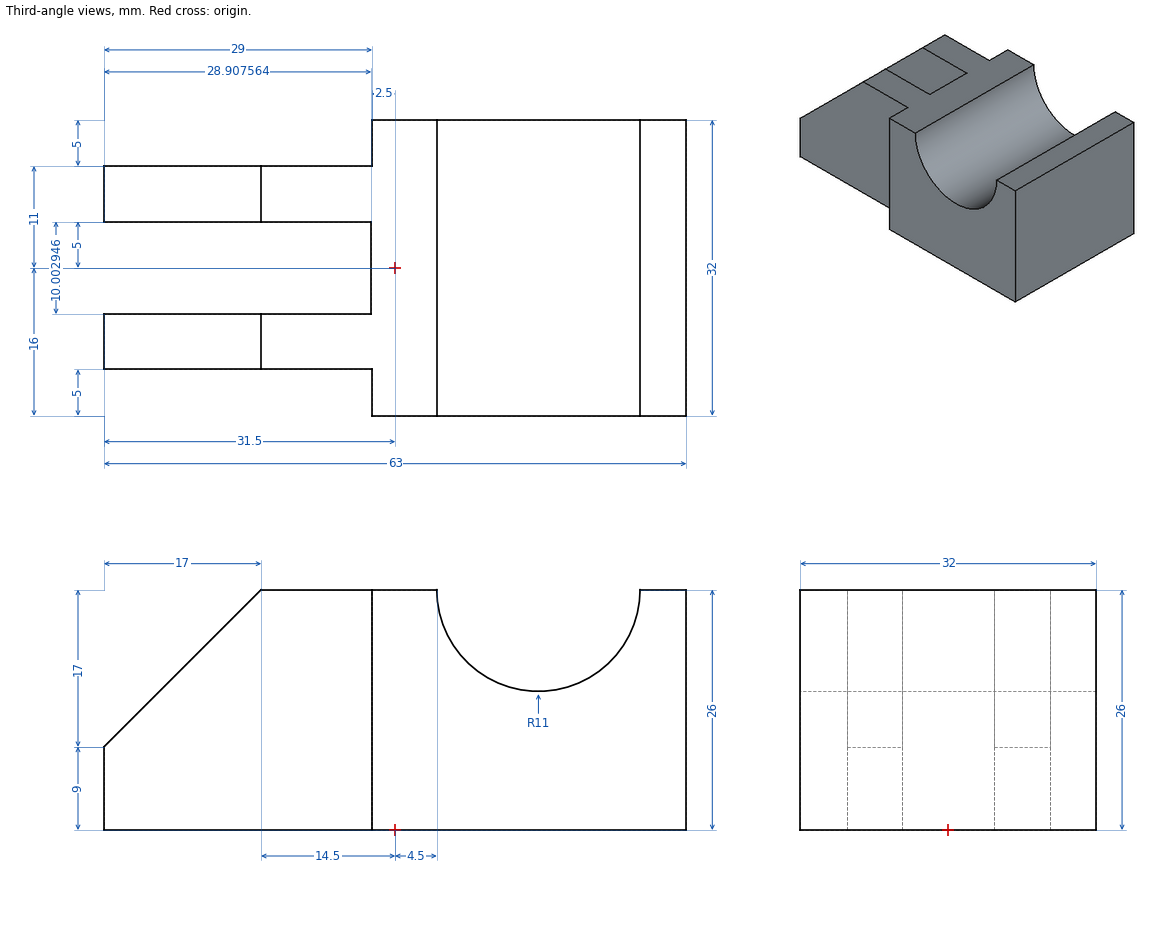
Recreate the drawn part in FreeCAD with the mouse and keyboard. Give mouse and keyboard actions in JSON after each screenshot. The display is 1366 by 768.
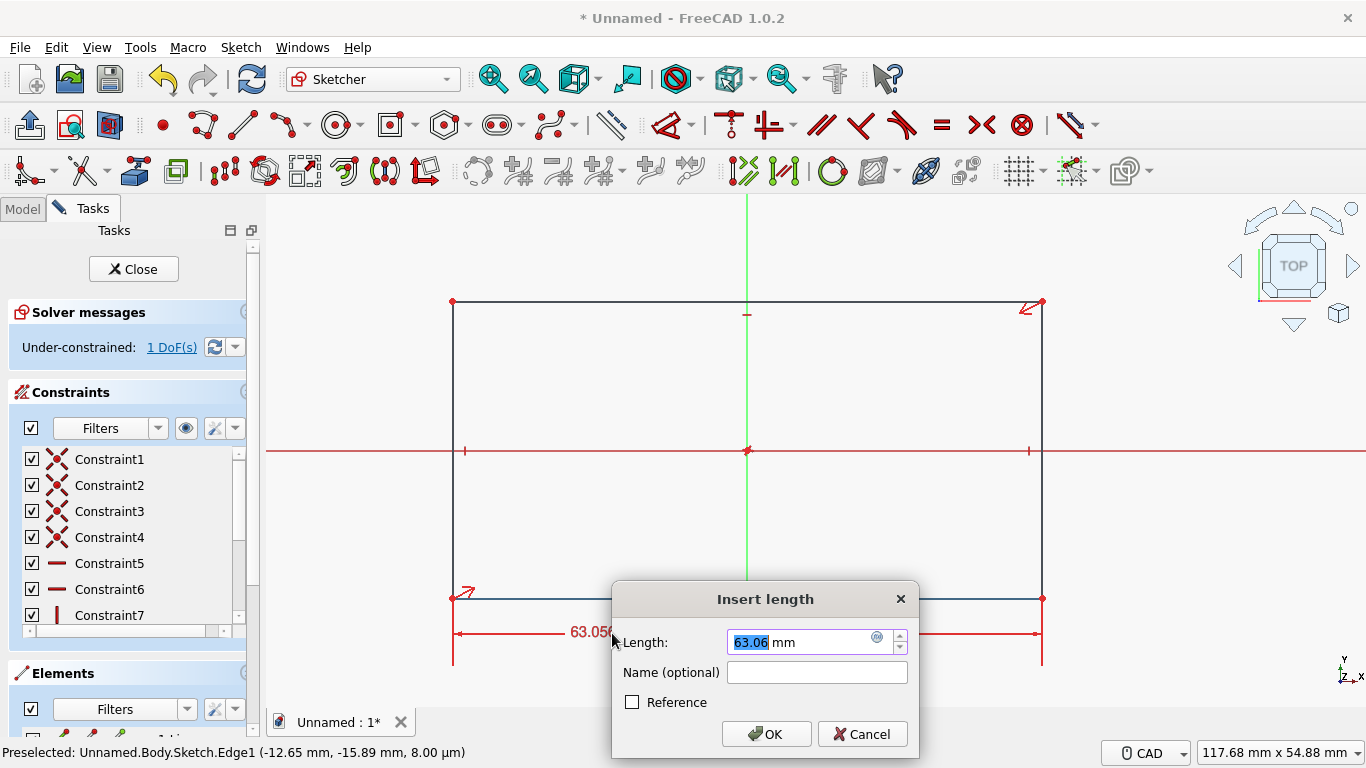
{"action": "type", "text": "63"}
{"action": "key", "text": "Return"}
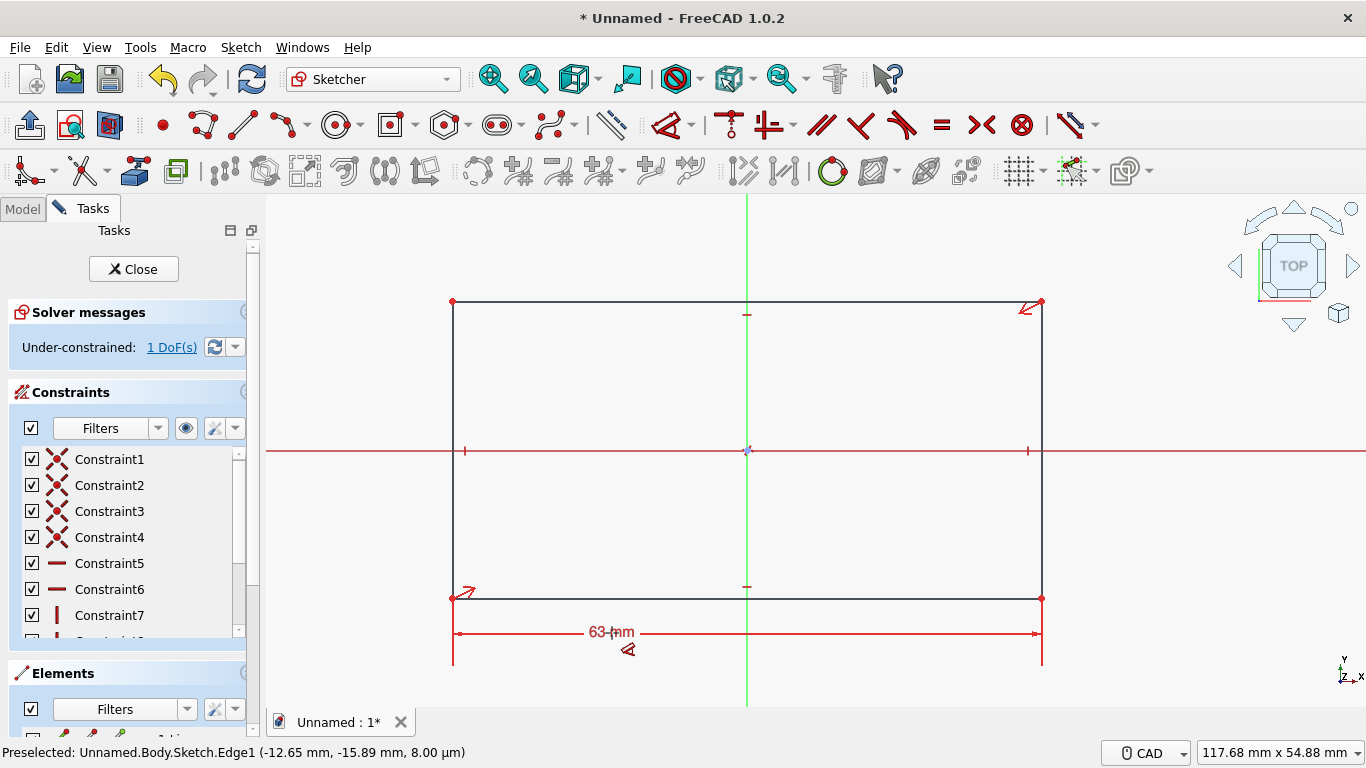
{"action": "left_click", "coordinate": [1042, 510]}
{"action": "left_click", "coordinate": [1076, 382]}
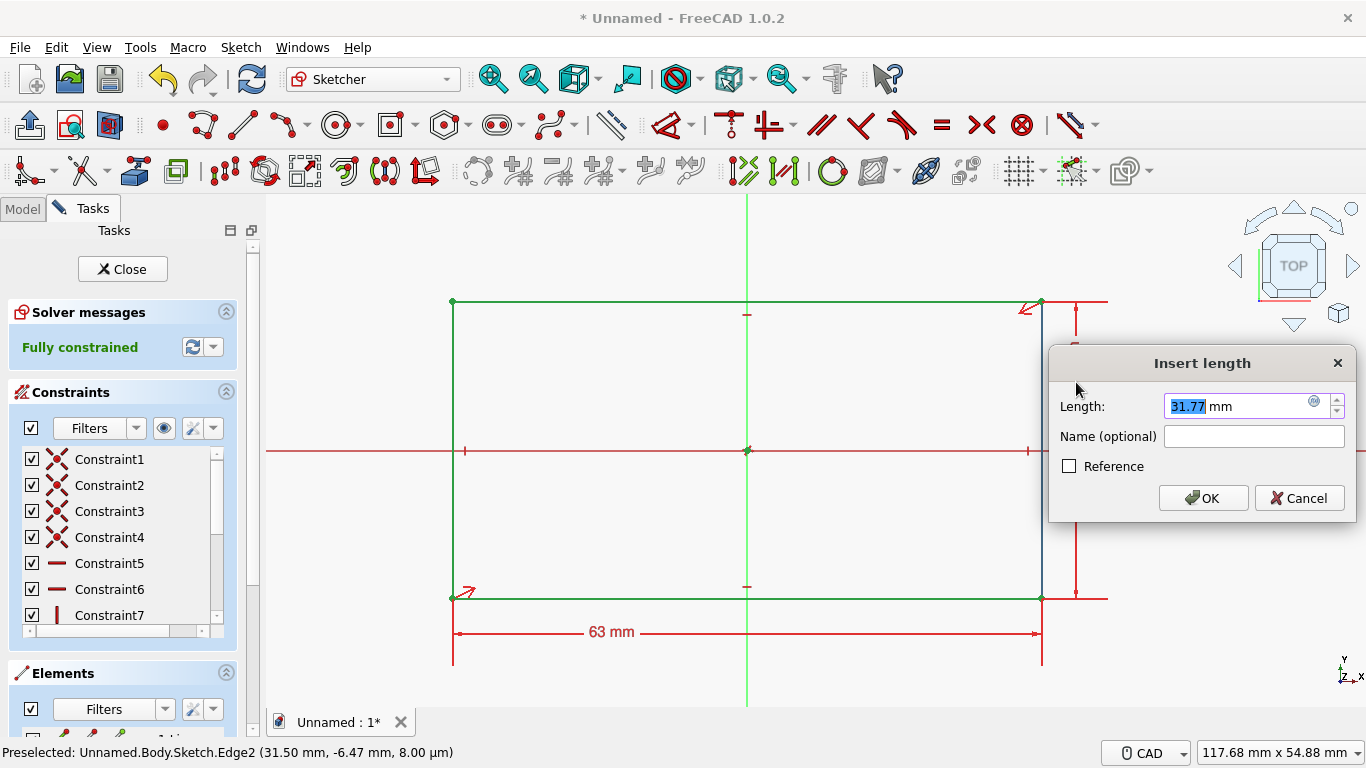
{"action": "type", "text": "32"}
{"action": "key", "text": "Return"}
{"action": "key", "text": "Escape"}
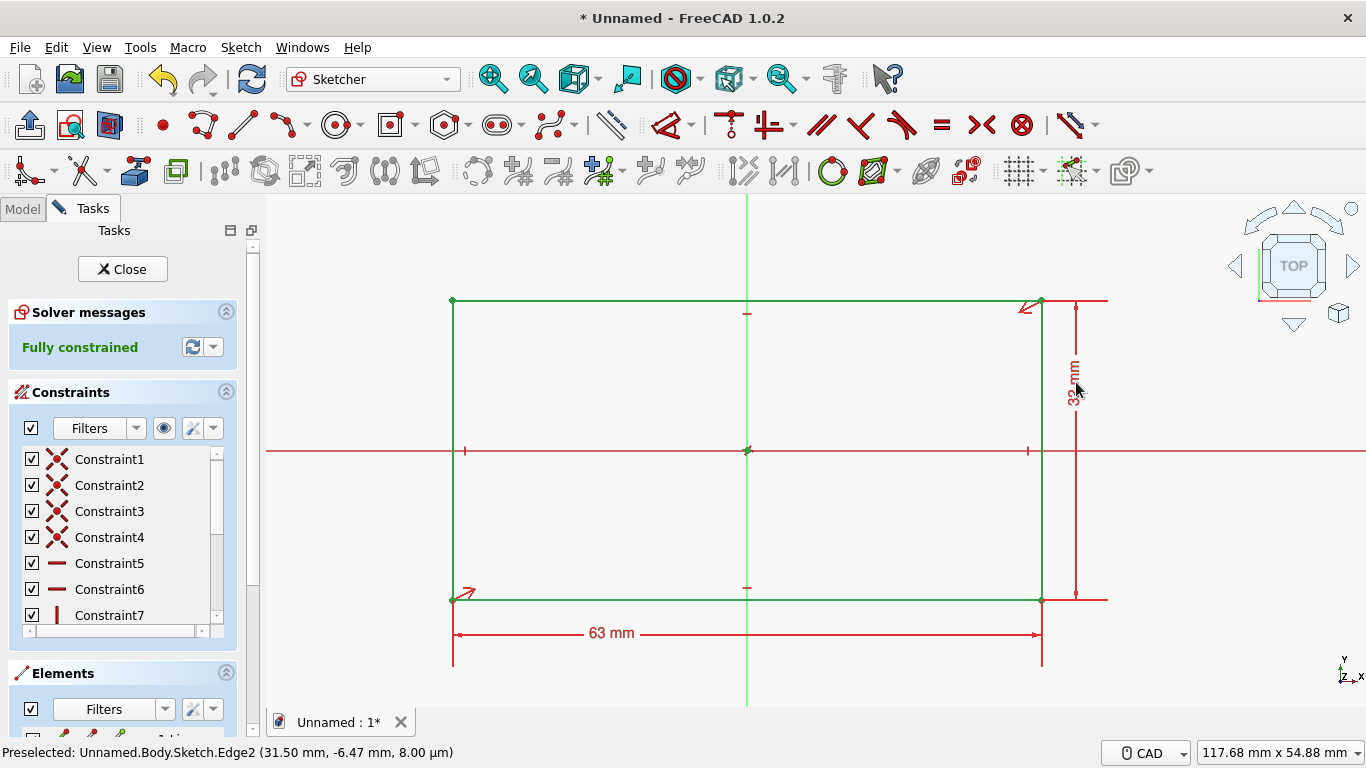
{"action": "left_click", "coordinate": [123, 269]}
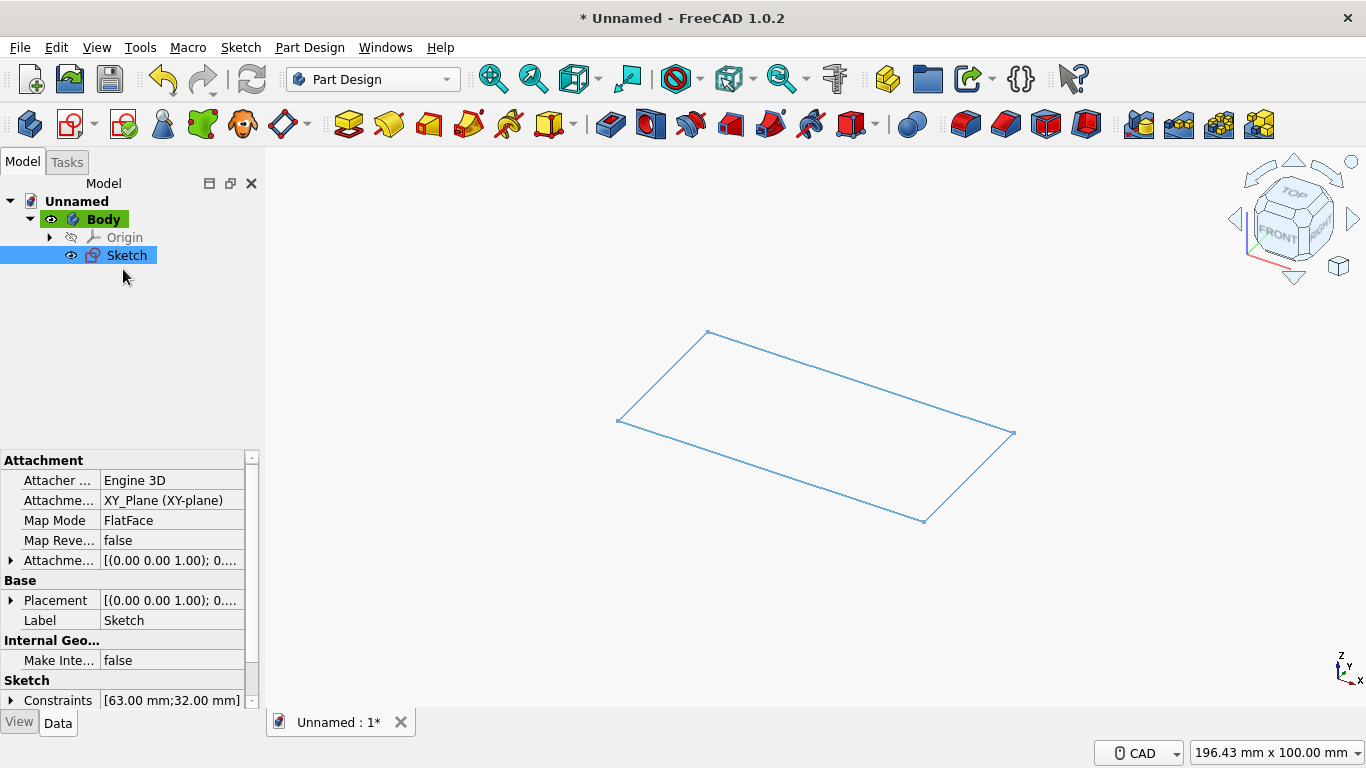
{"action": "left_click", "coordinate": [350, 124]}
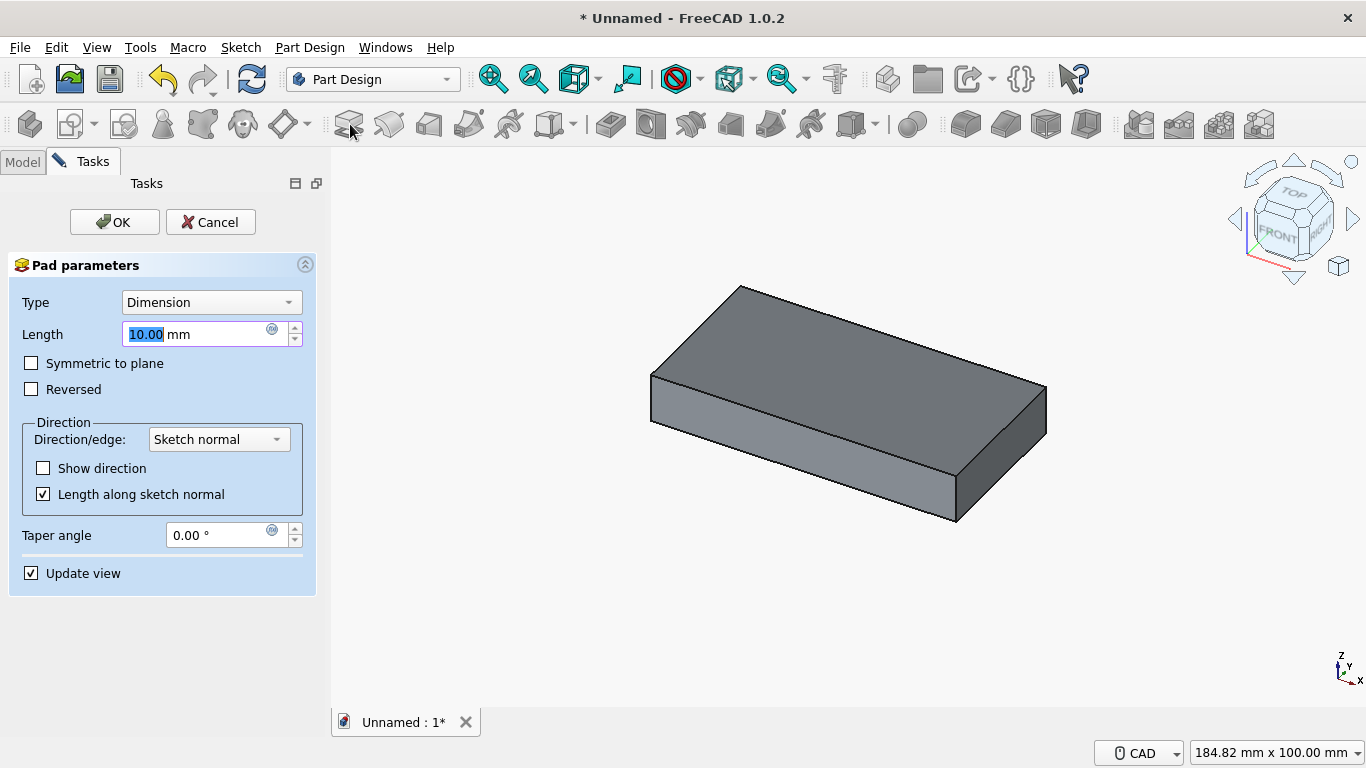
{"action": "type", "text": "26"}
{"action": "key", "text": "Tab"}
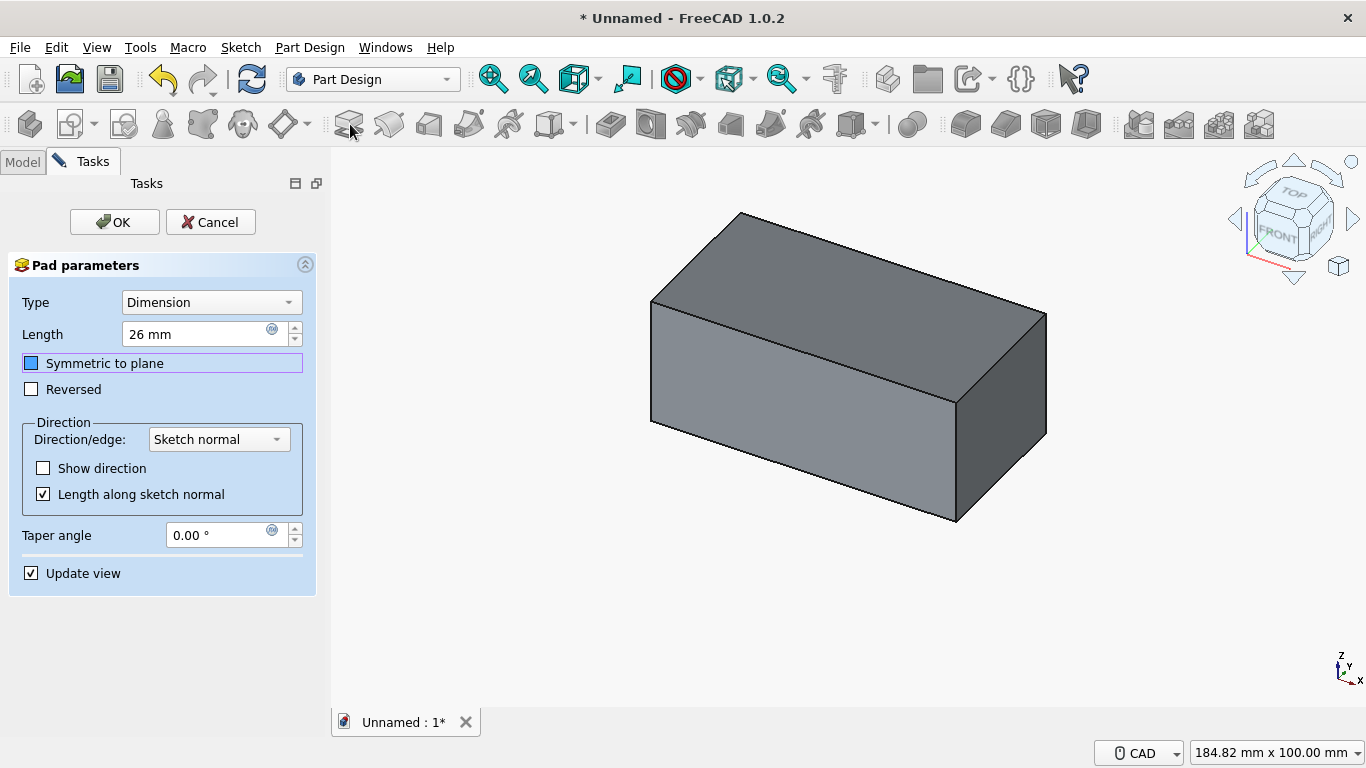
{"action": "left_click", "coordinate": [115, 222]}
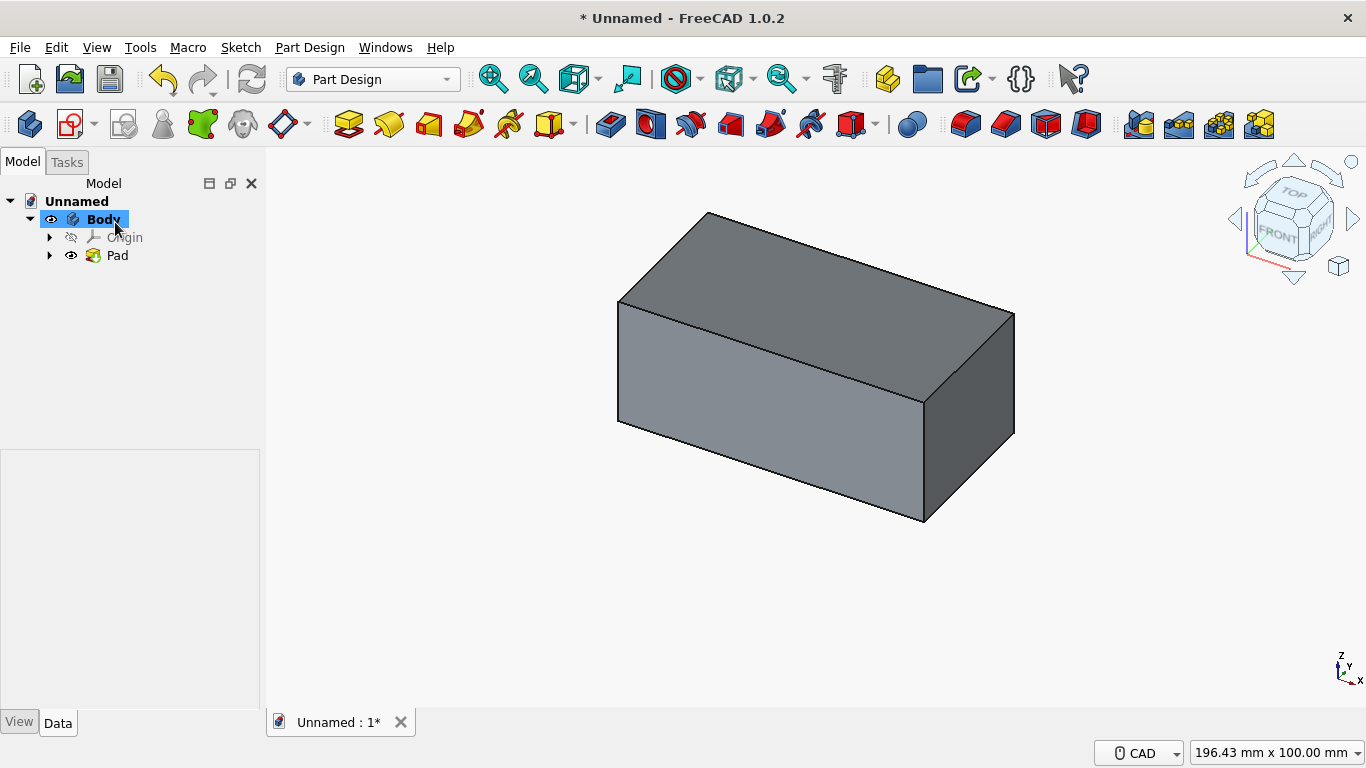
{"action": "left_click", "coordinate": [858, 440]}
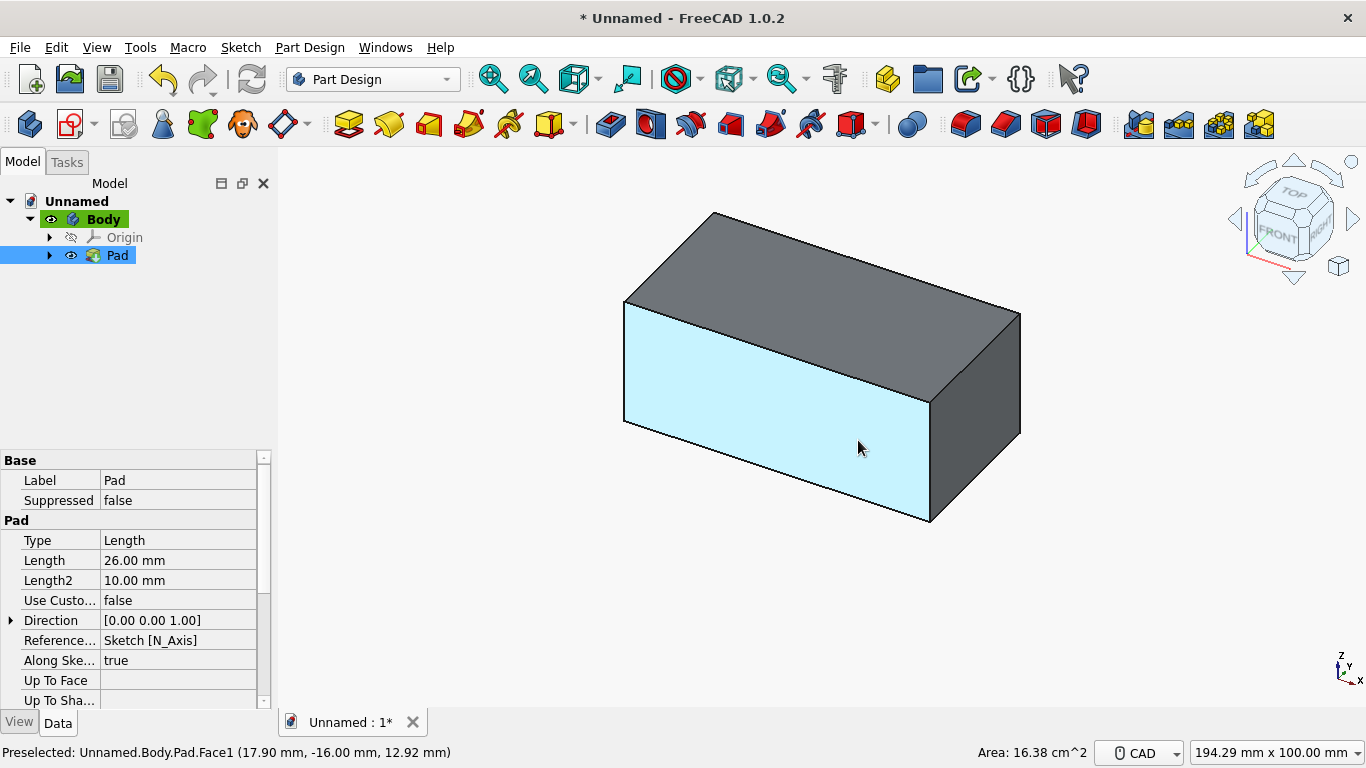
{"action": "left_click", "coordinate": [70, 124]}